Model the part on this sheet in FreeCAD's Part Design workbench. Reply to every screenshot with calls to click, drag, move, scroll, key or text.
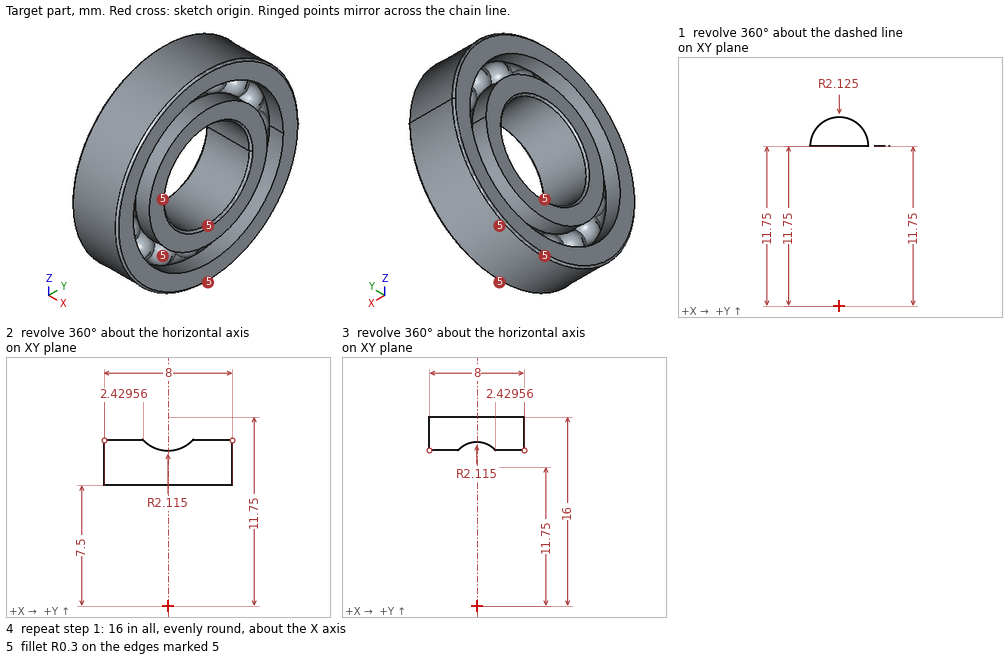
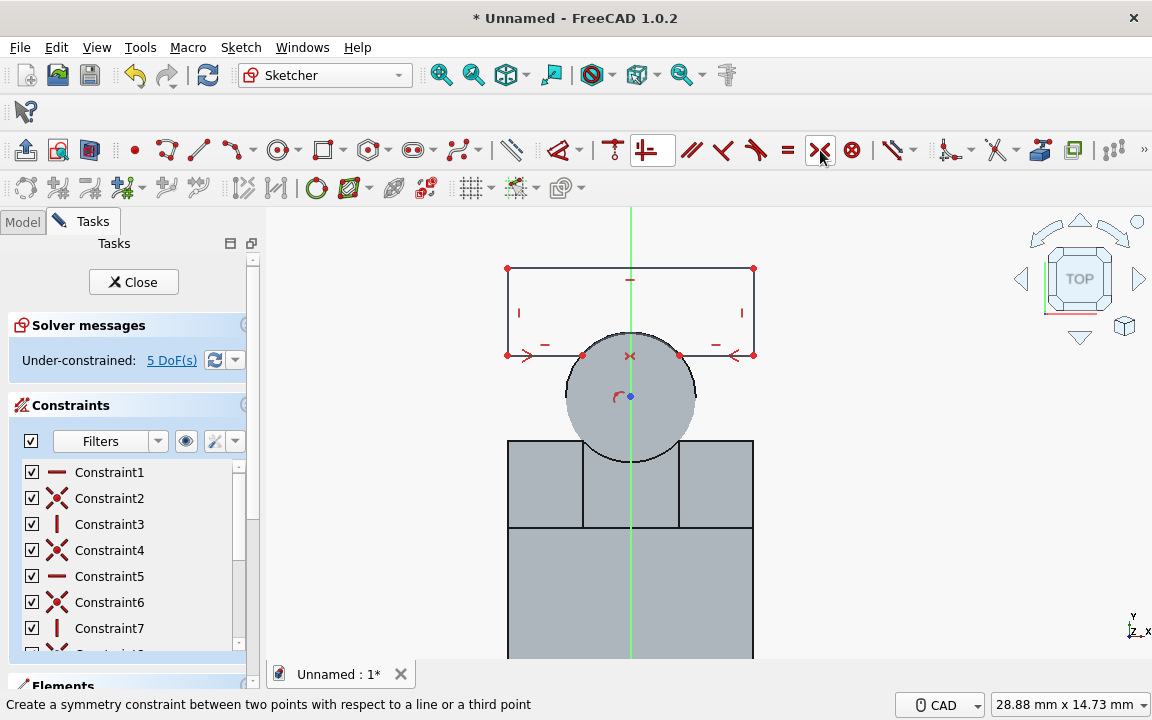
click(558, 150)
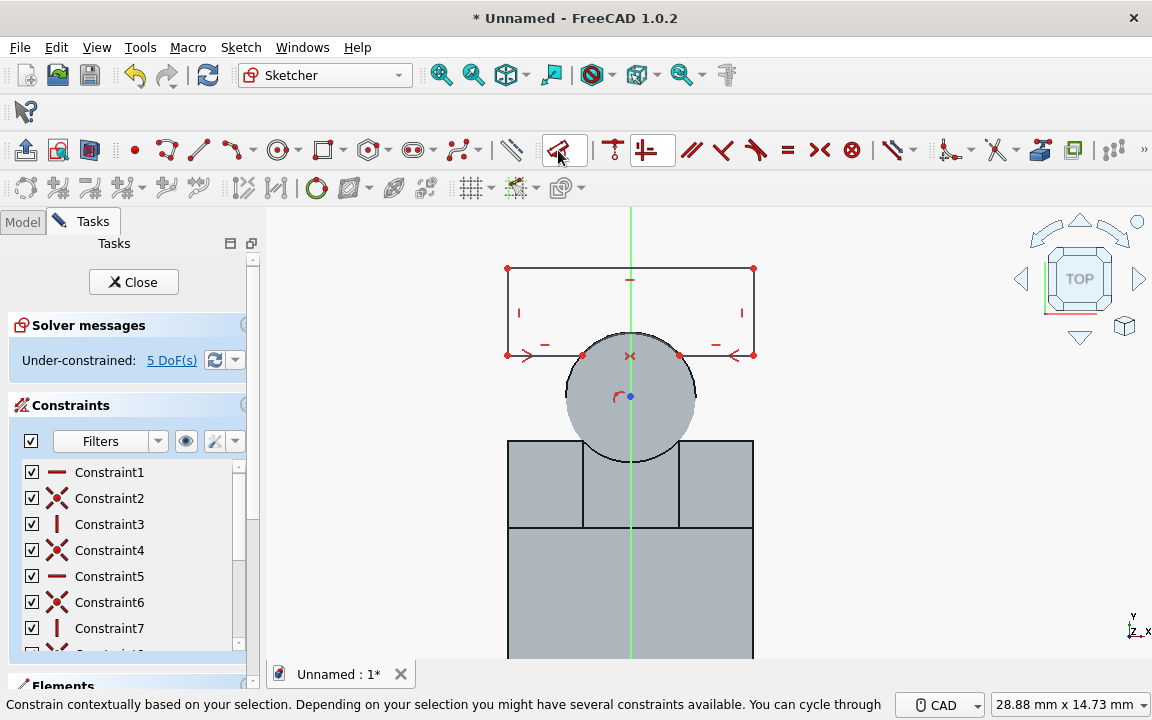
click(652, 337)
click(663, 307)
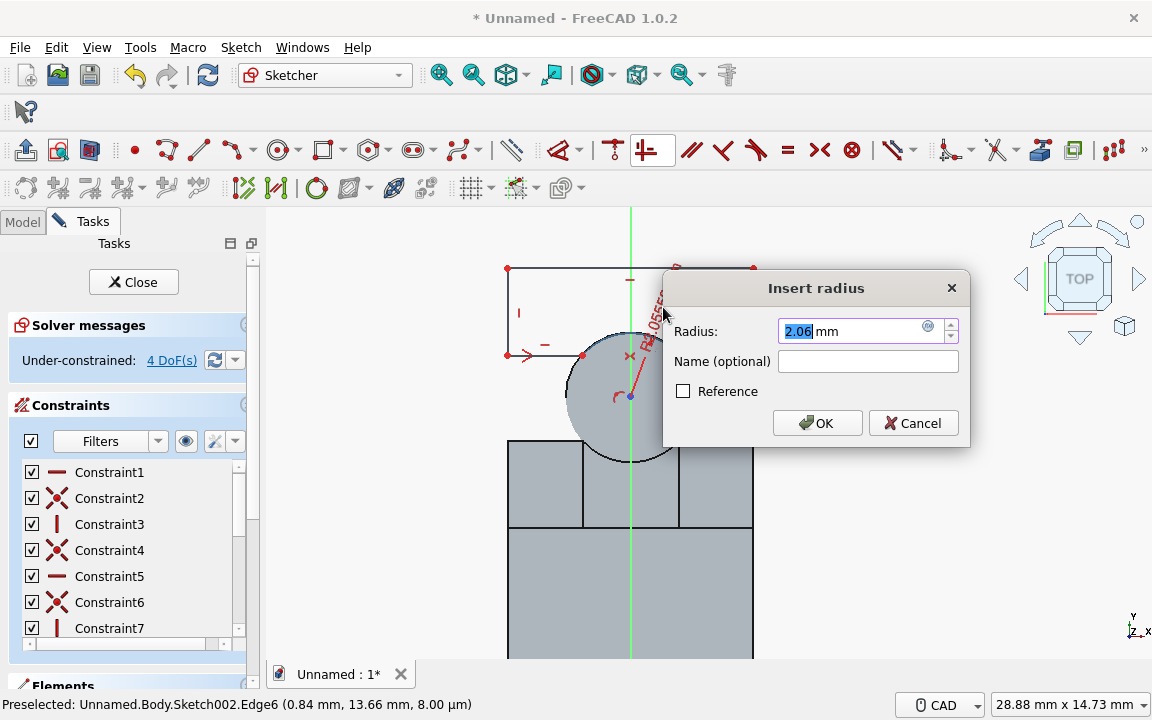
text(2.115)
key(Return)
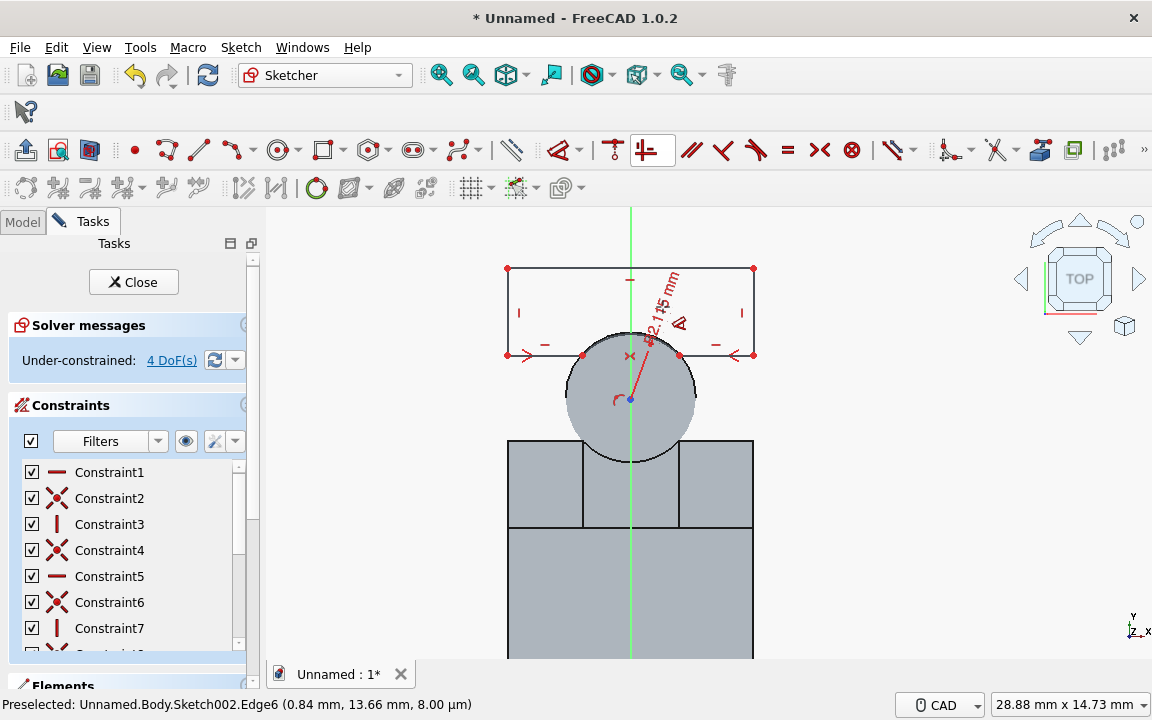
click(680, 268)
click(574, 302)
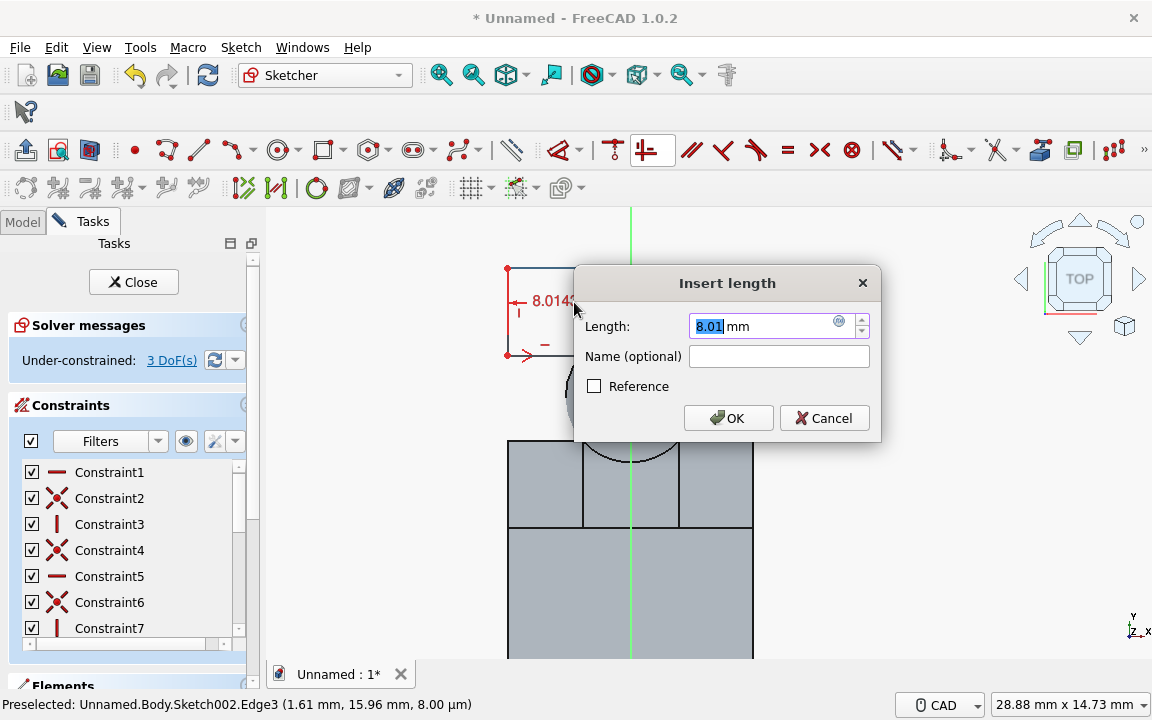
text(8)
key(Return)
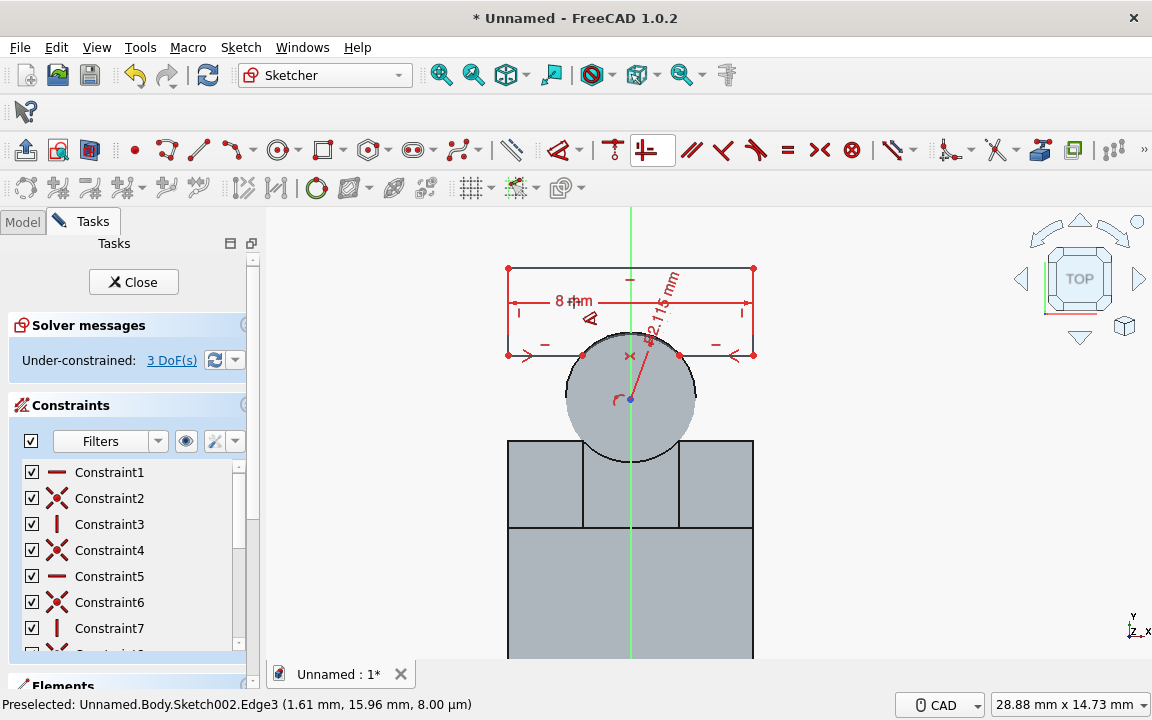
click(753, 268)
click(787, 450)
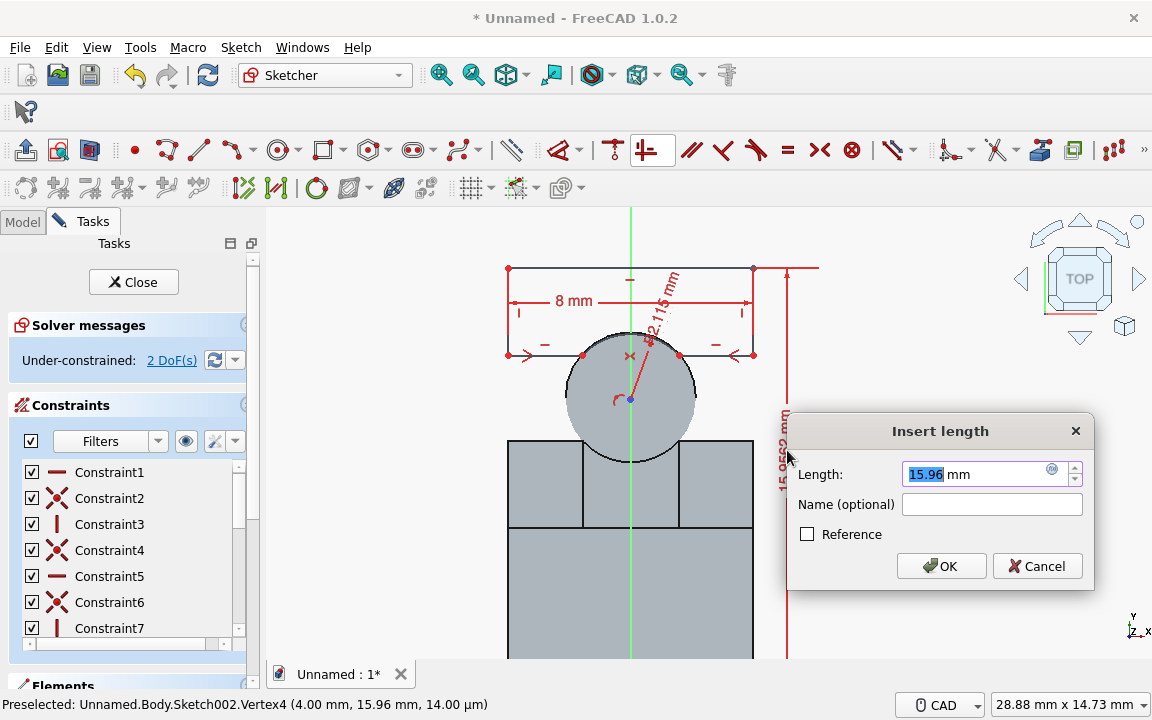
text(16)
key(Return)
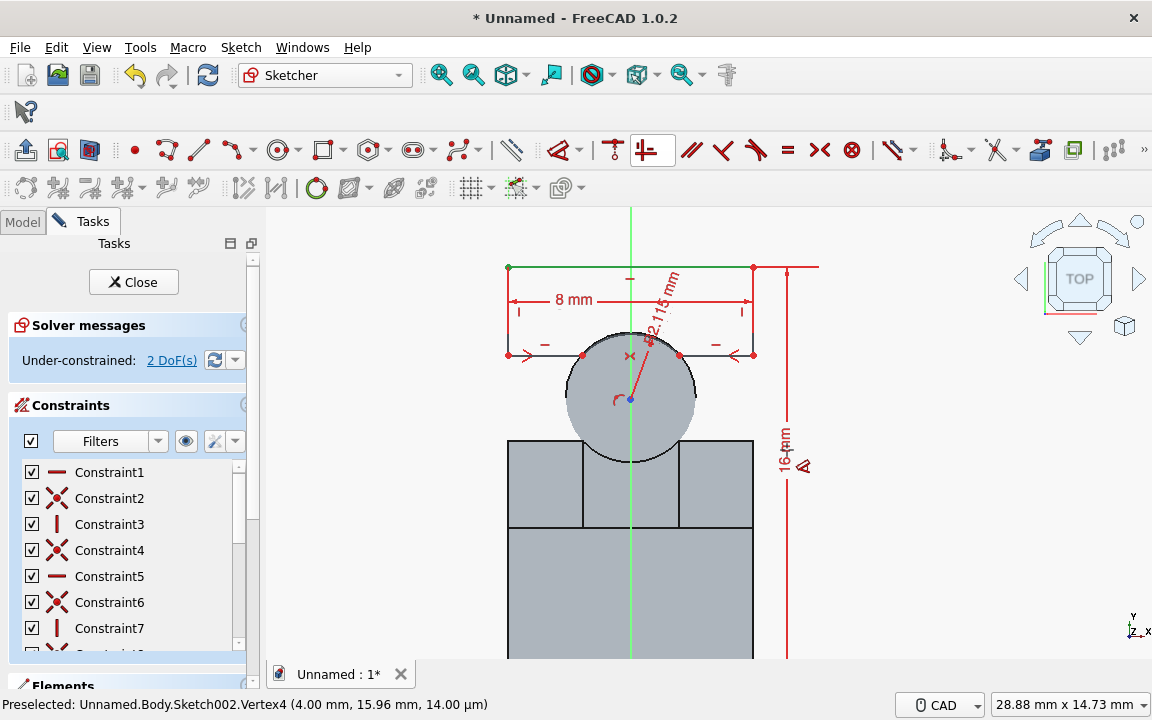
click(631, 399)
click(665, 515)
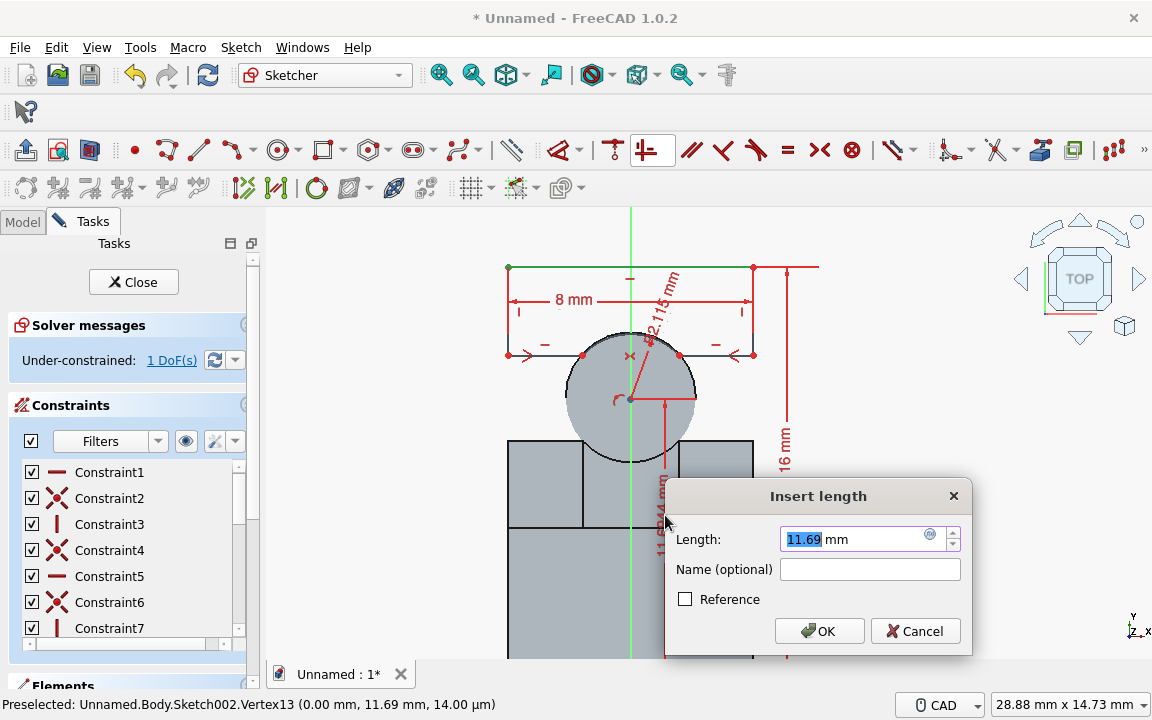
text(11.75)
key(Return)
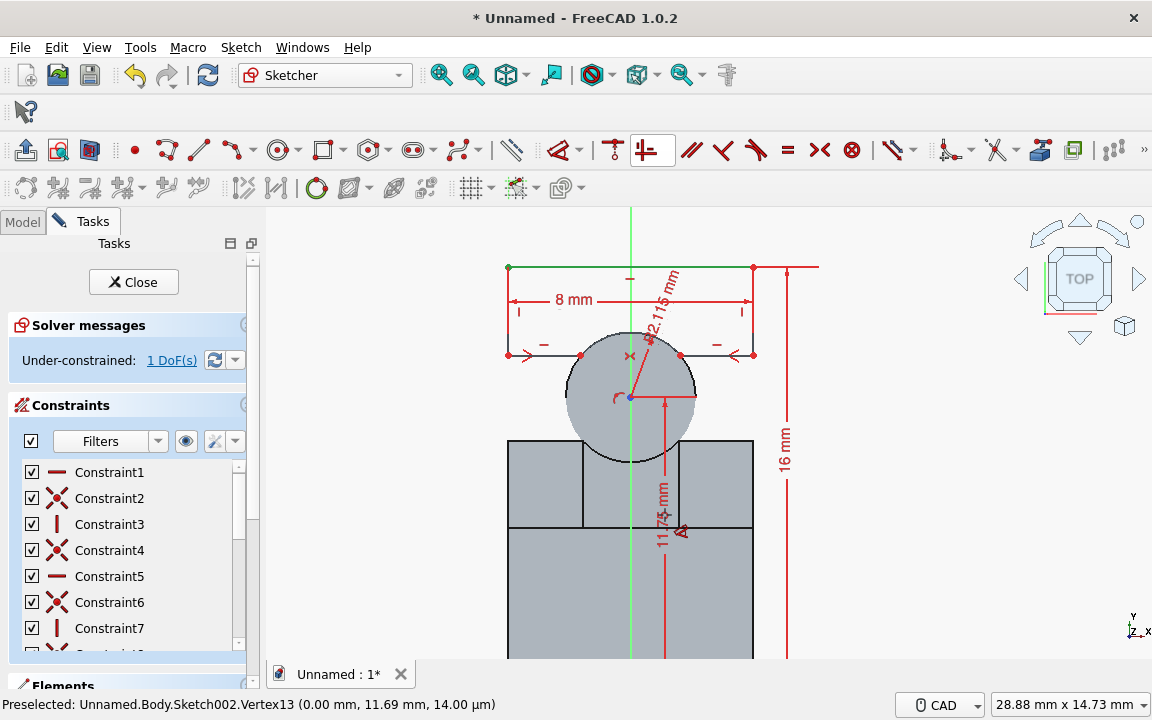
click(702, 356)
click(734, 322)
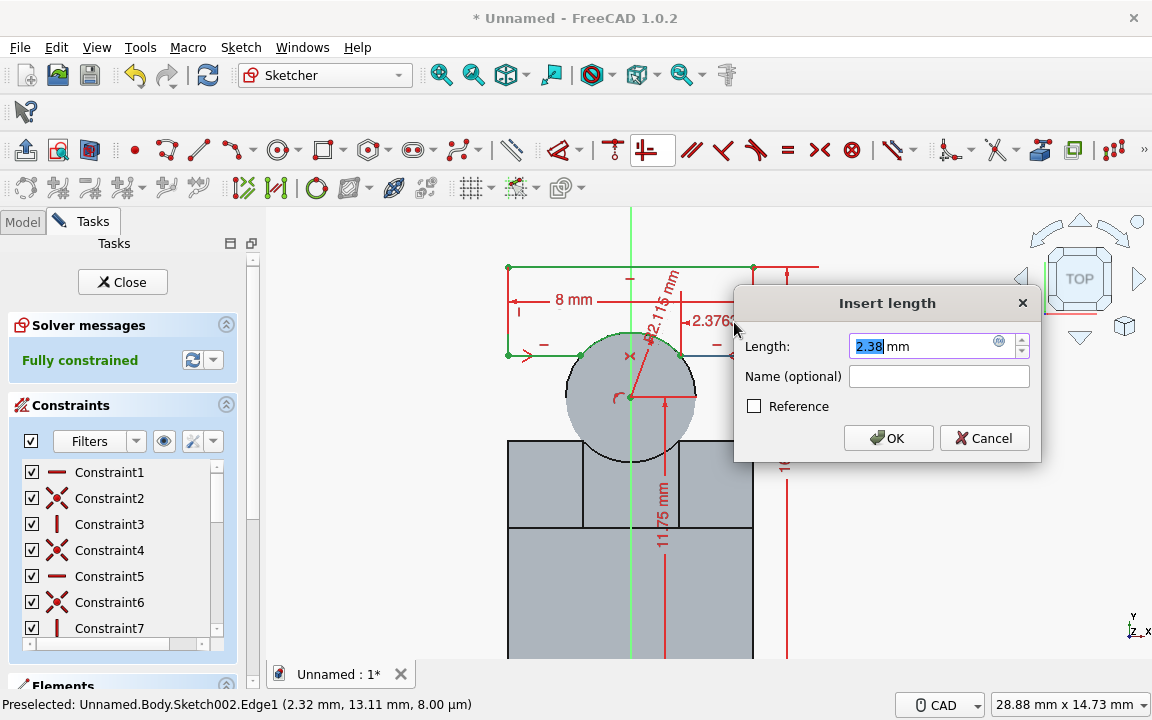
text(2.42956)
key(Return)
key(Escape)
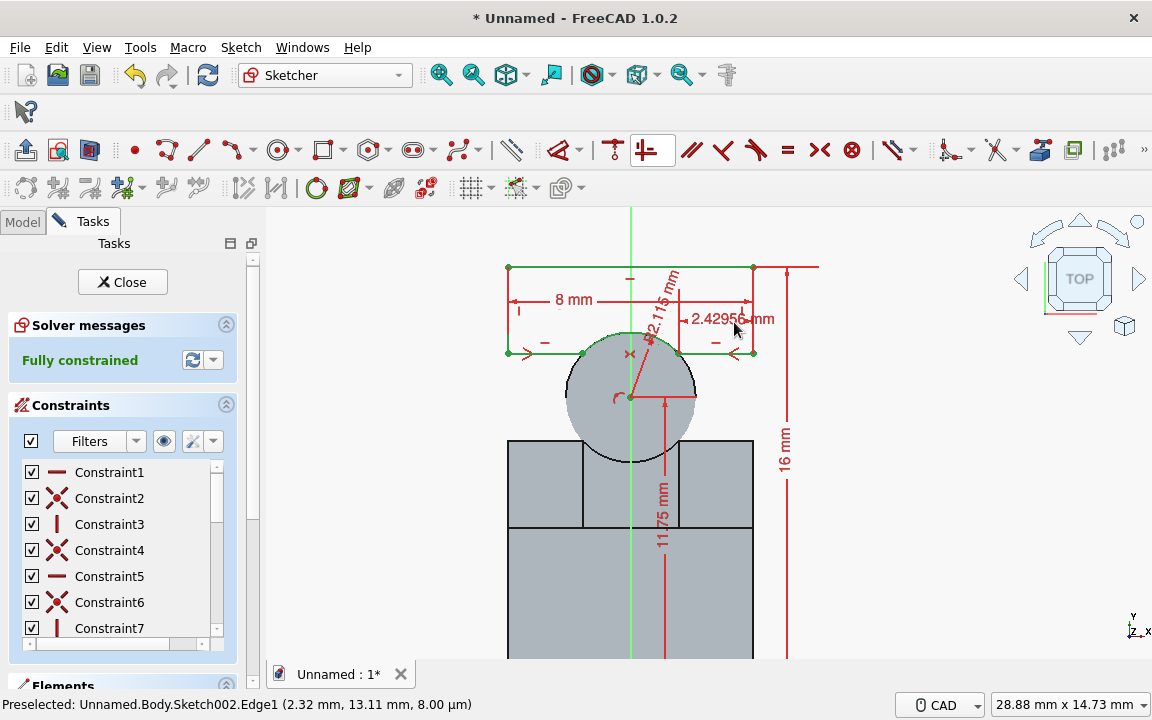
click(123, 282)